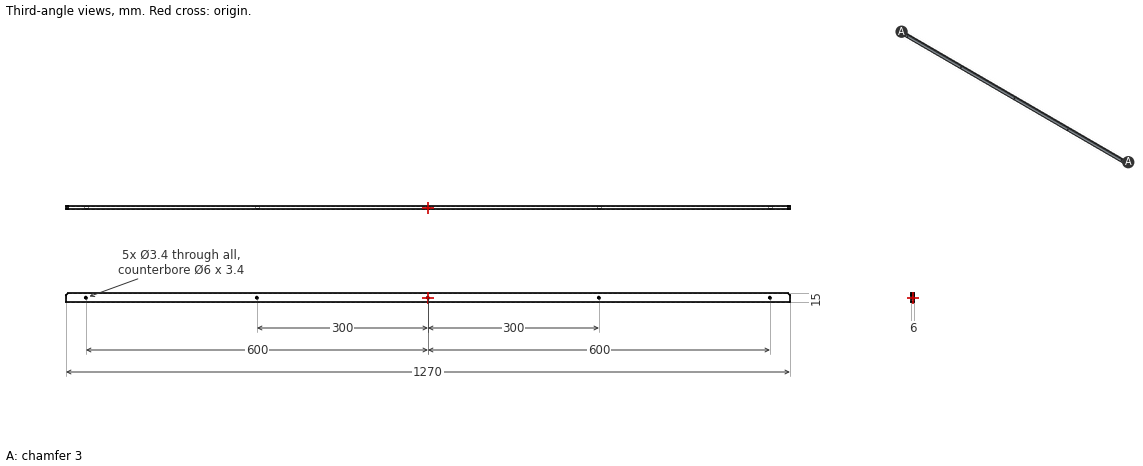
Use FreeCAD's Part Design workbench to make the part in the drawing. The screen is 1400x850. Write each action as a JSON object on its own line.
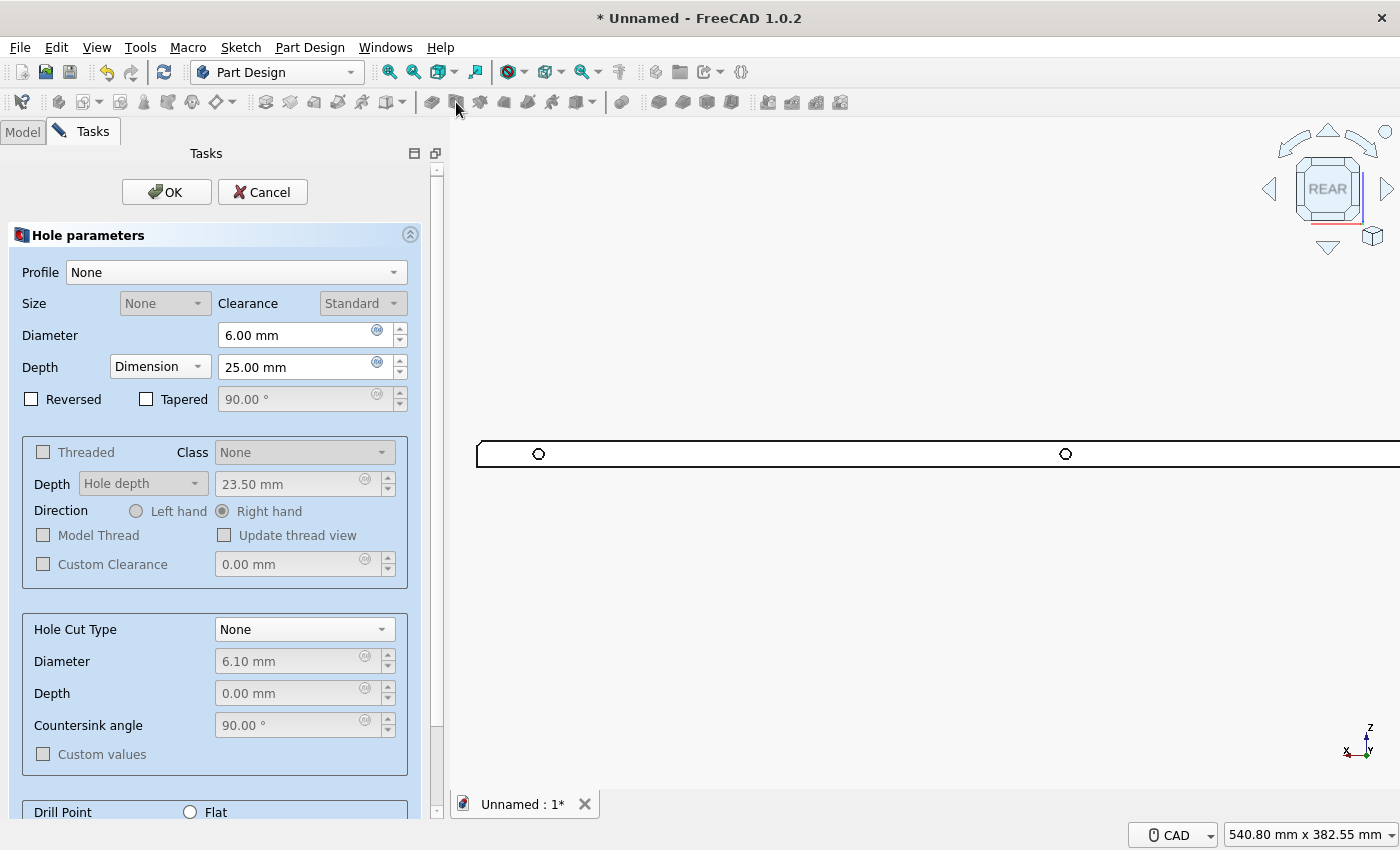
{"action": "triple_click", "coordinate": [305, 335]}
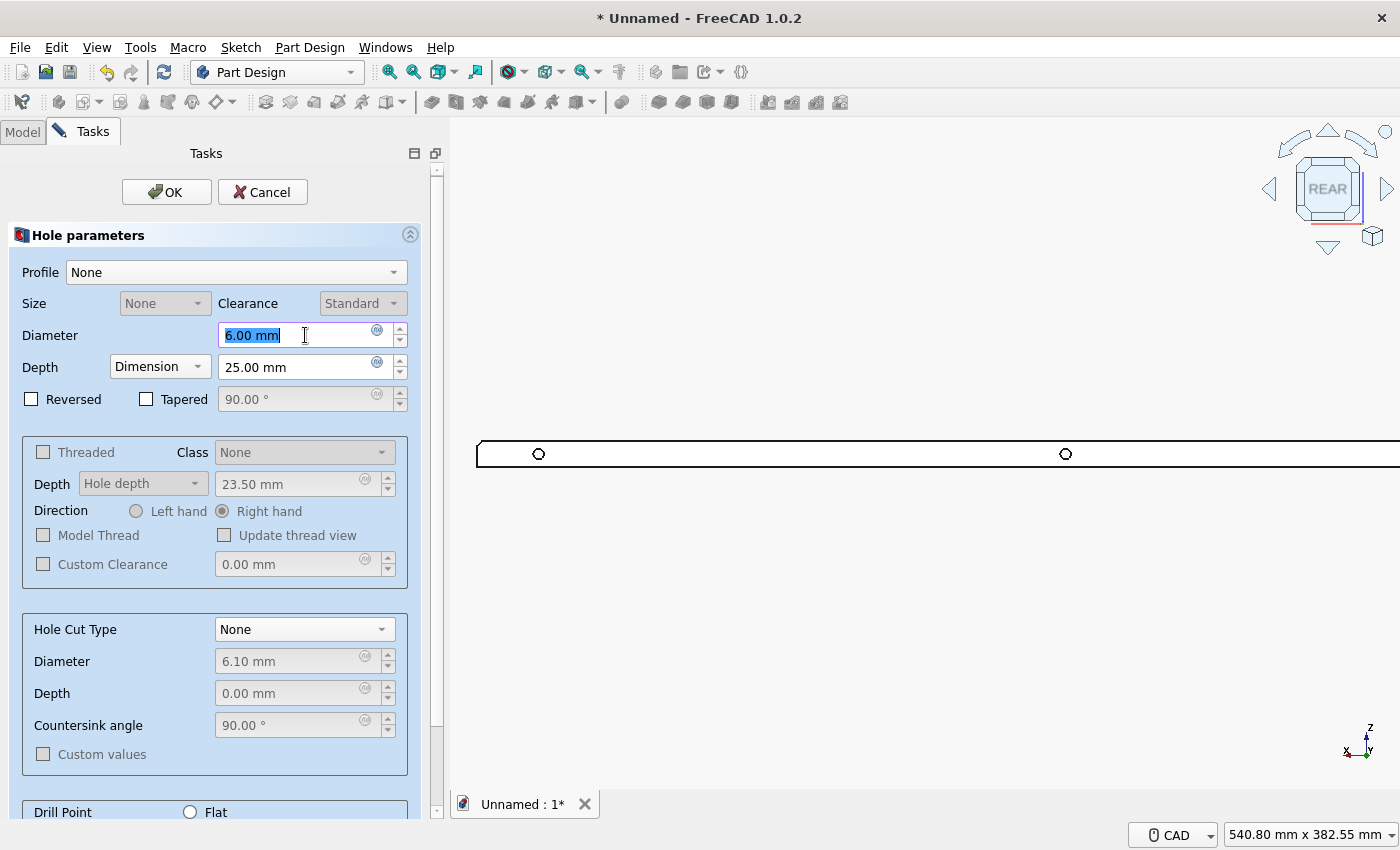
{"action": "type", "text": "3.4"}
{"action": "key", "text": "Tab"}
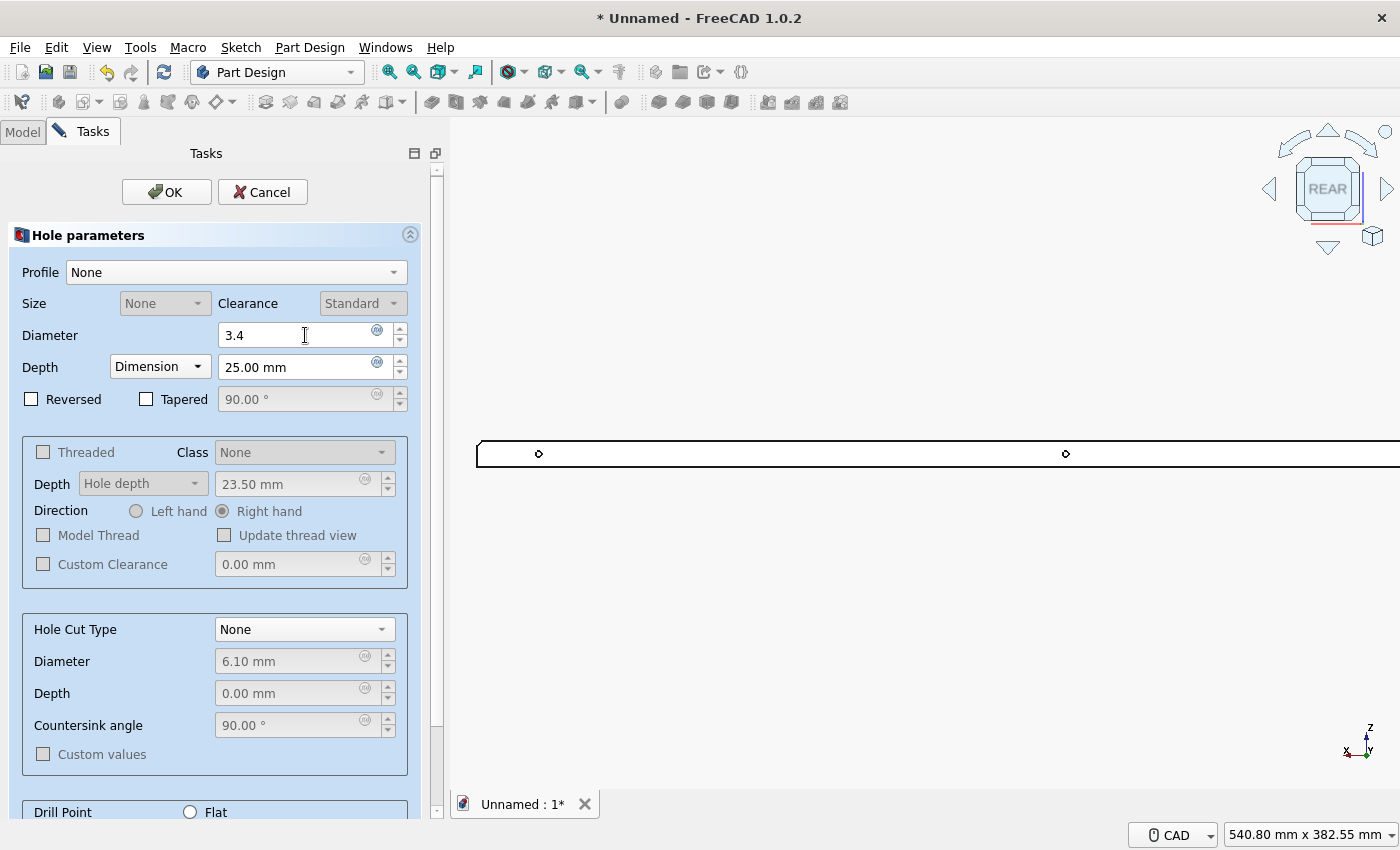
{"action": "left_click", "coordinate": [161, 366]}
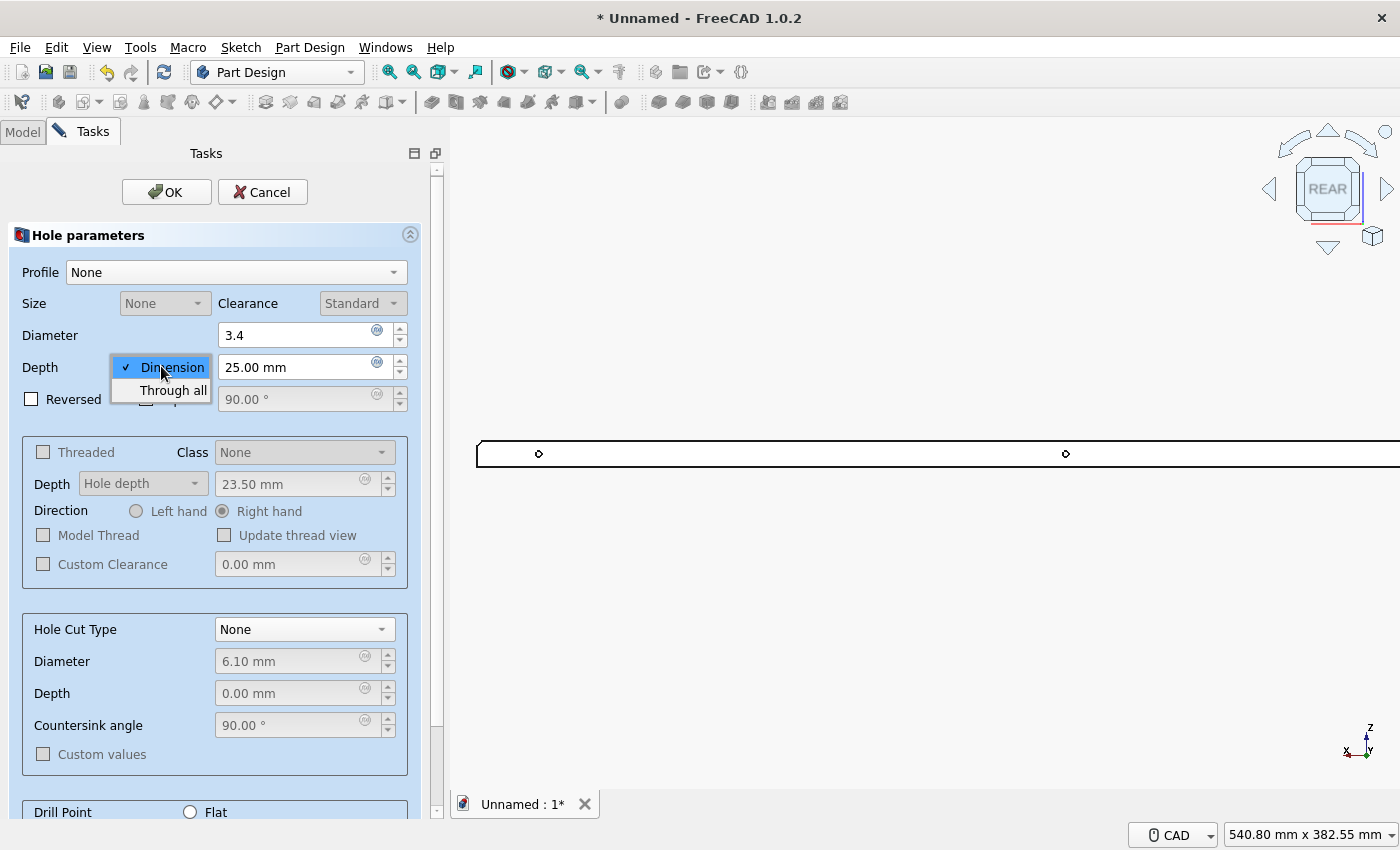
{"action": "left_click", "coordinate": [160, 390]}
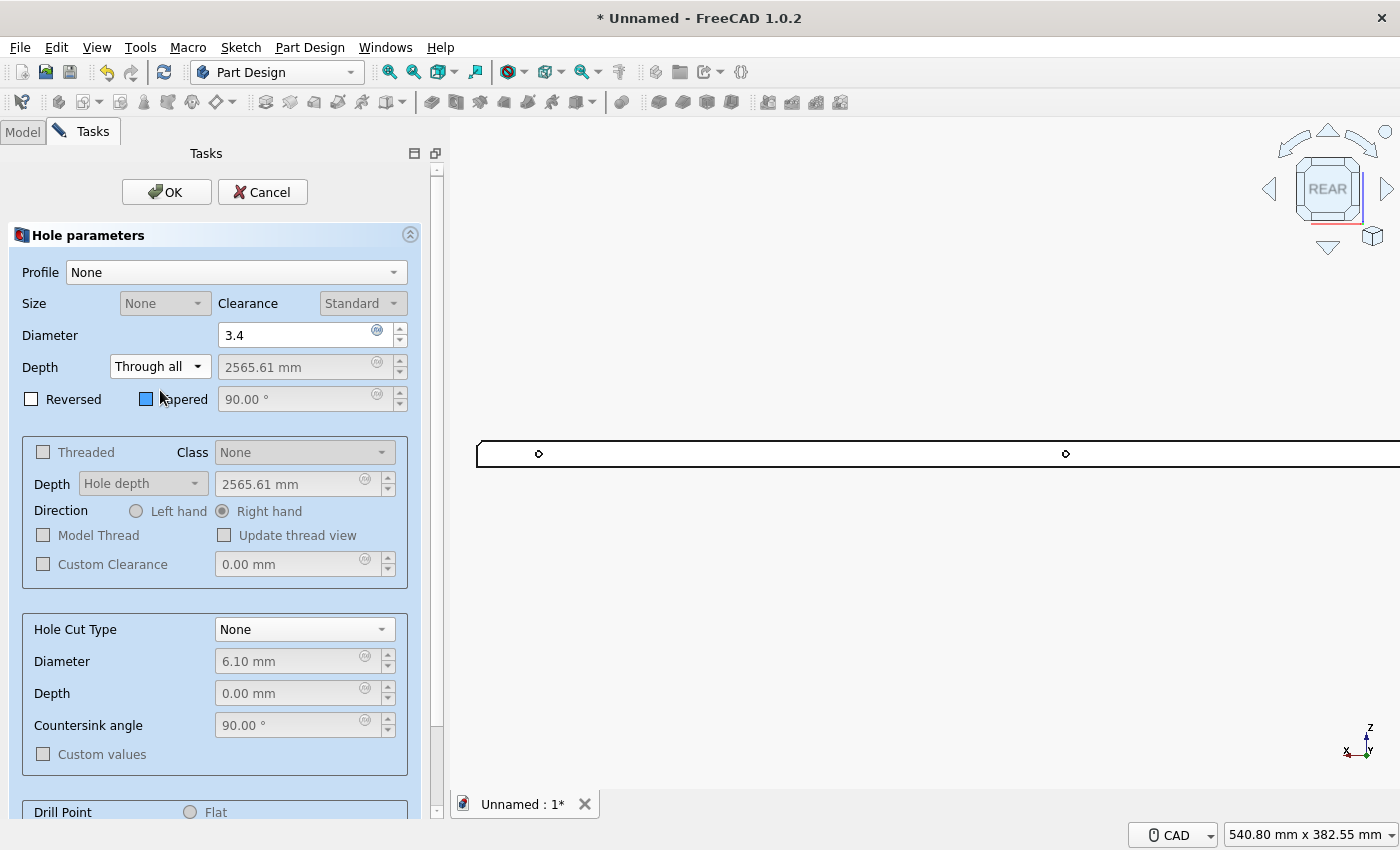
{"action": "left_click", "coordinate": [306, 630]}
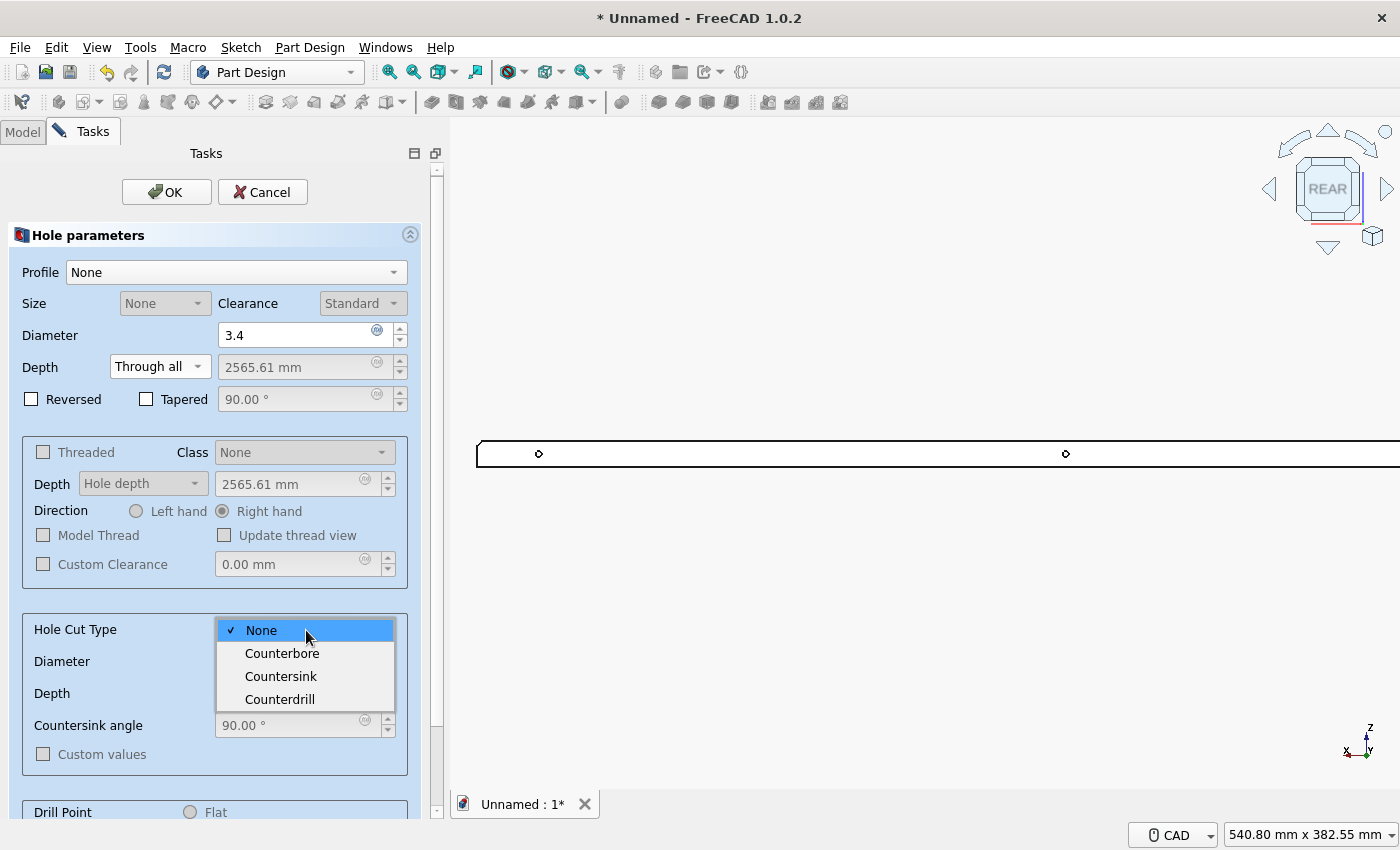
{"action": "left_click", "coordinate": [304, 654]}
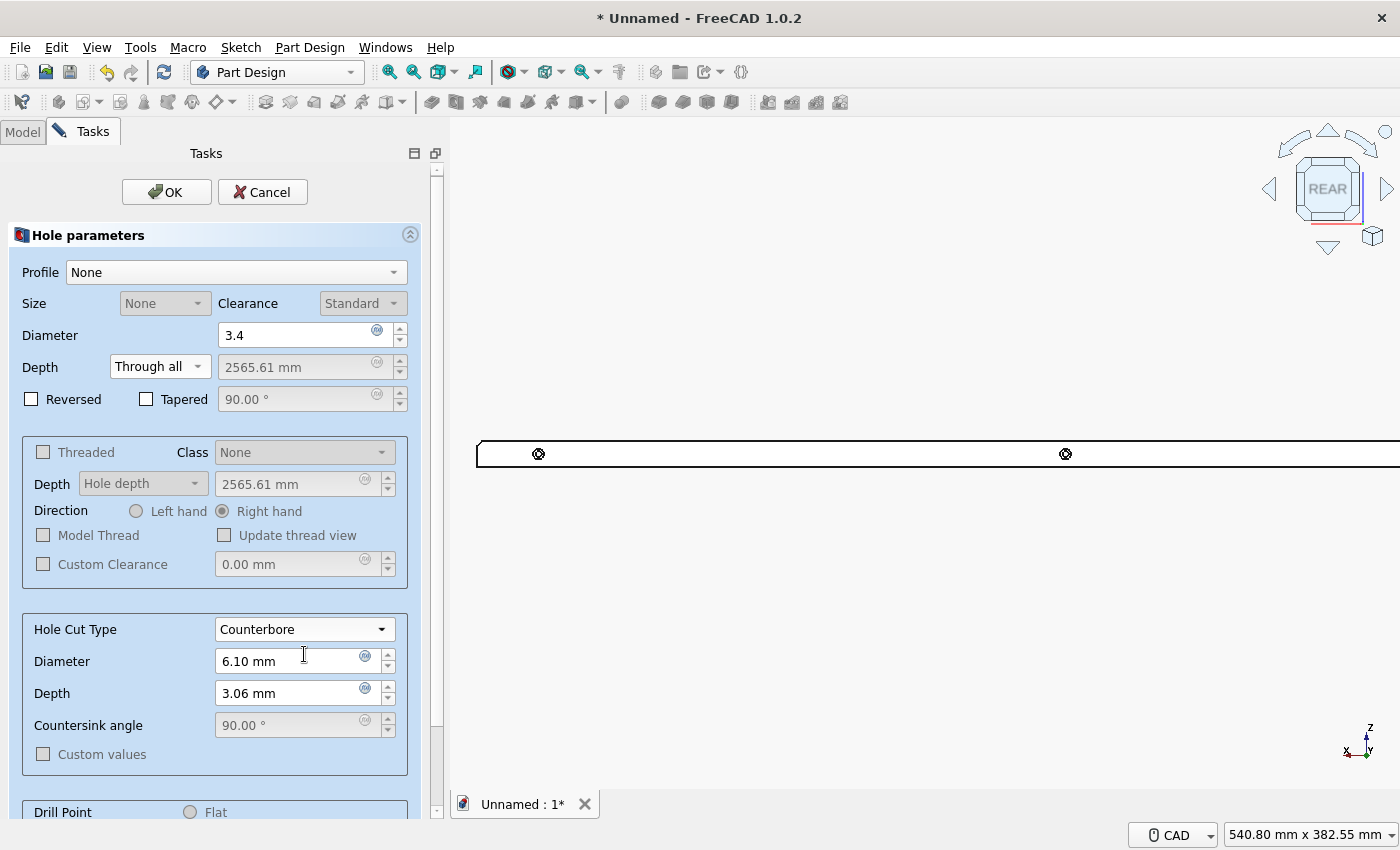
{"action": "triple_click", "coordinate": [298, 661]}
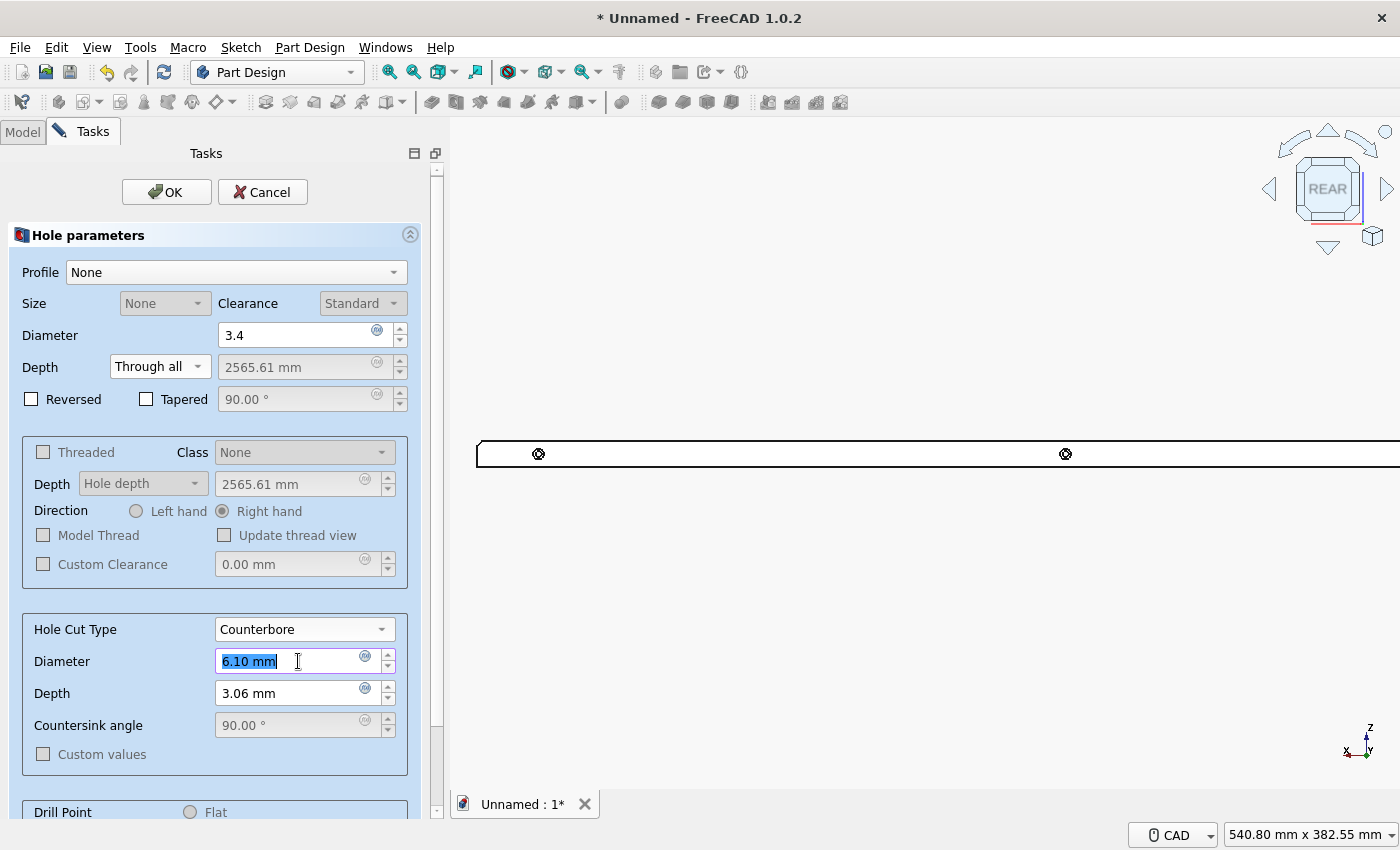
{"action": "type", "text": "6"}
{"action": "key", "text": "Tab"}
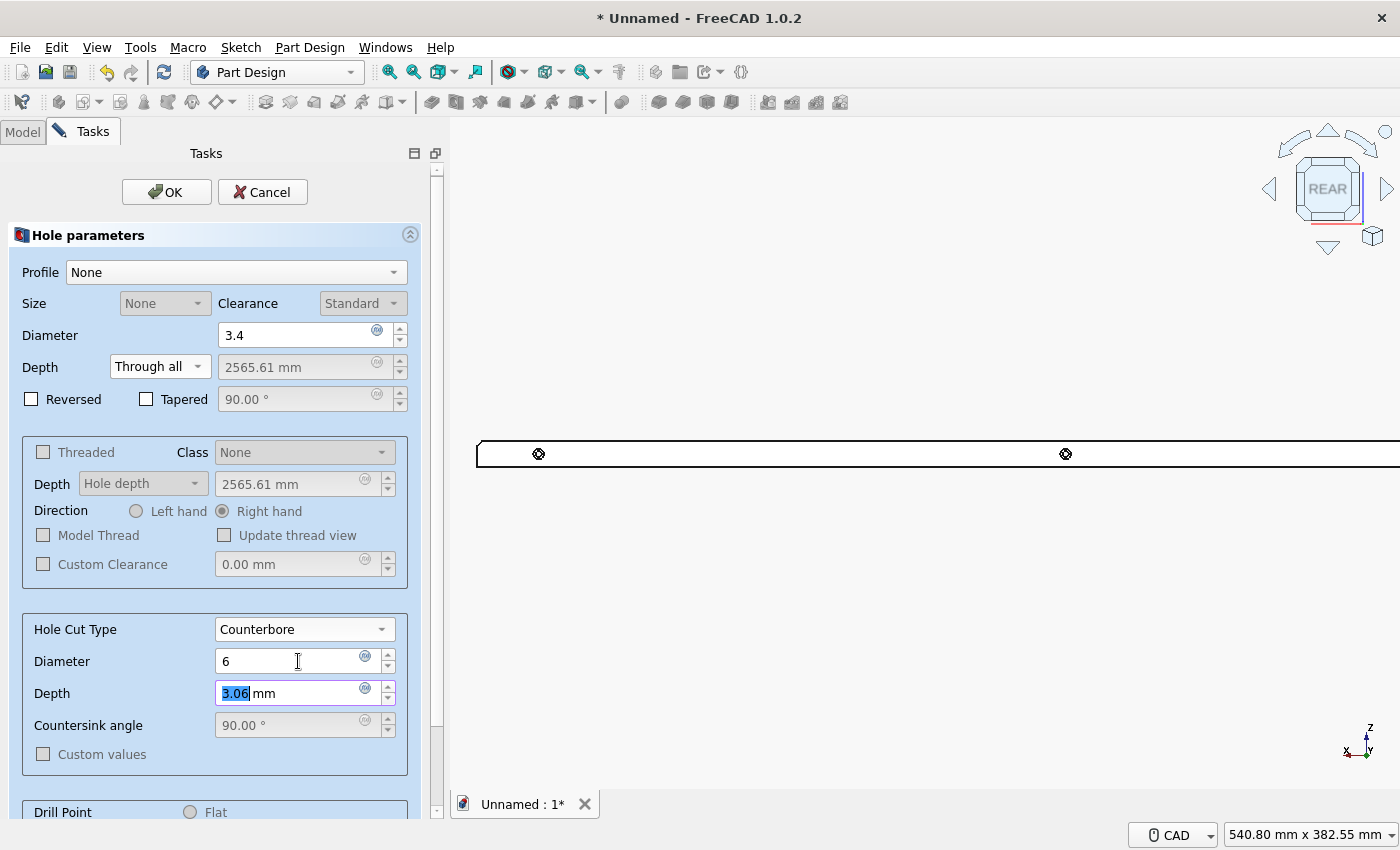
{"action": "type", "text": "3.4"}
{"action": "key", "text": "Tab"}